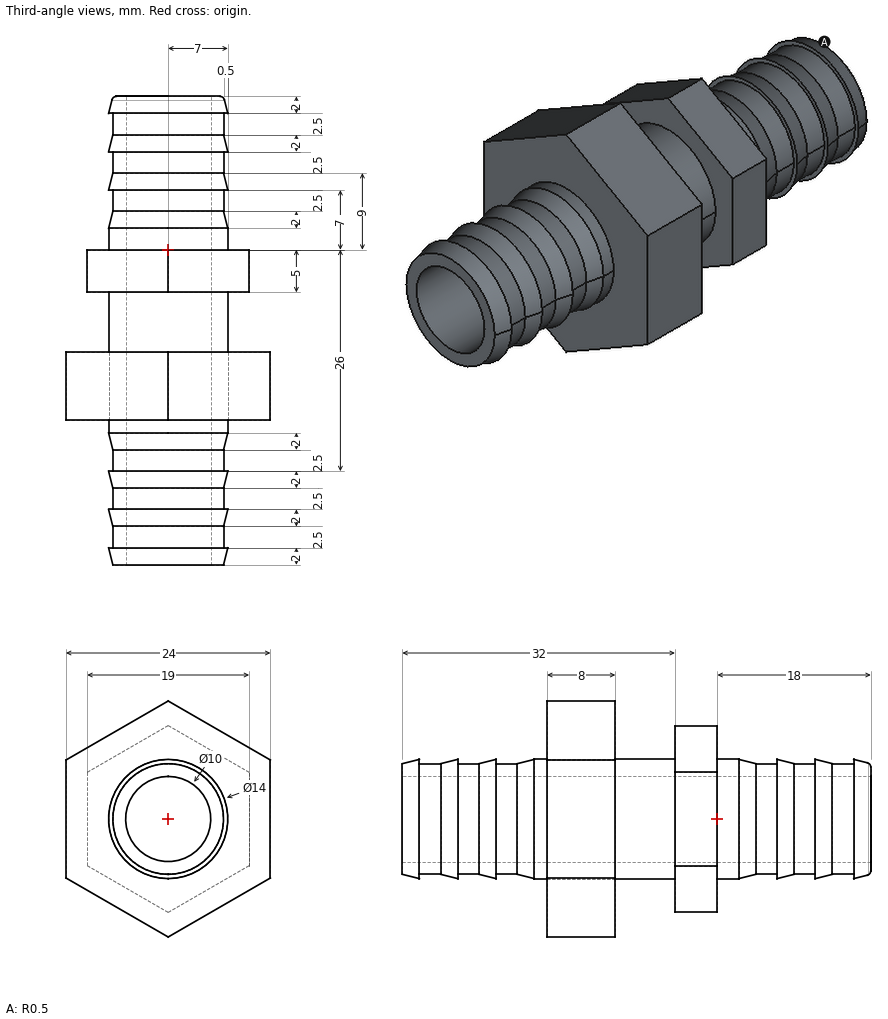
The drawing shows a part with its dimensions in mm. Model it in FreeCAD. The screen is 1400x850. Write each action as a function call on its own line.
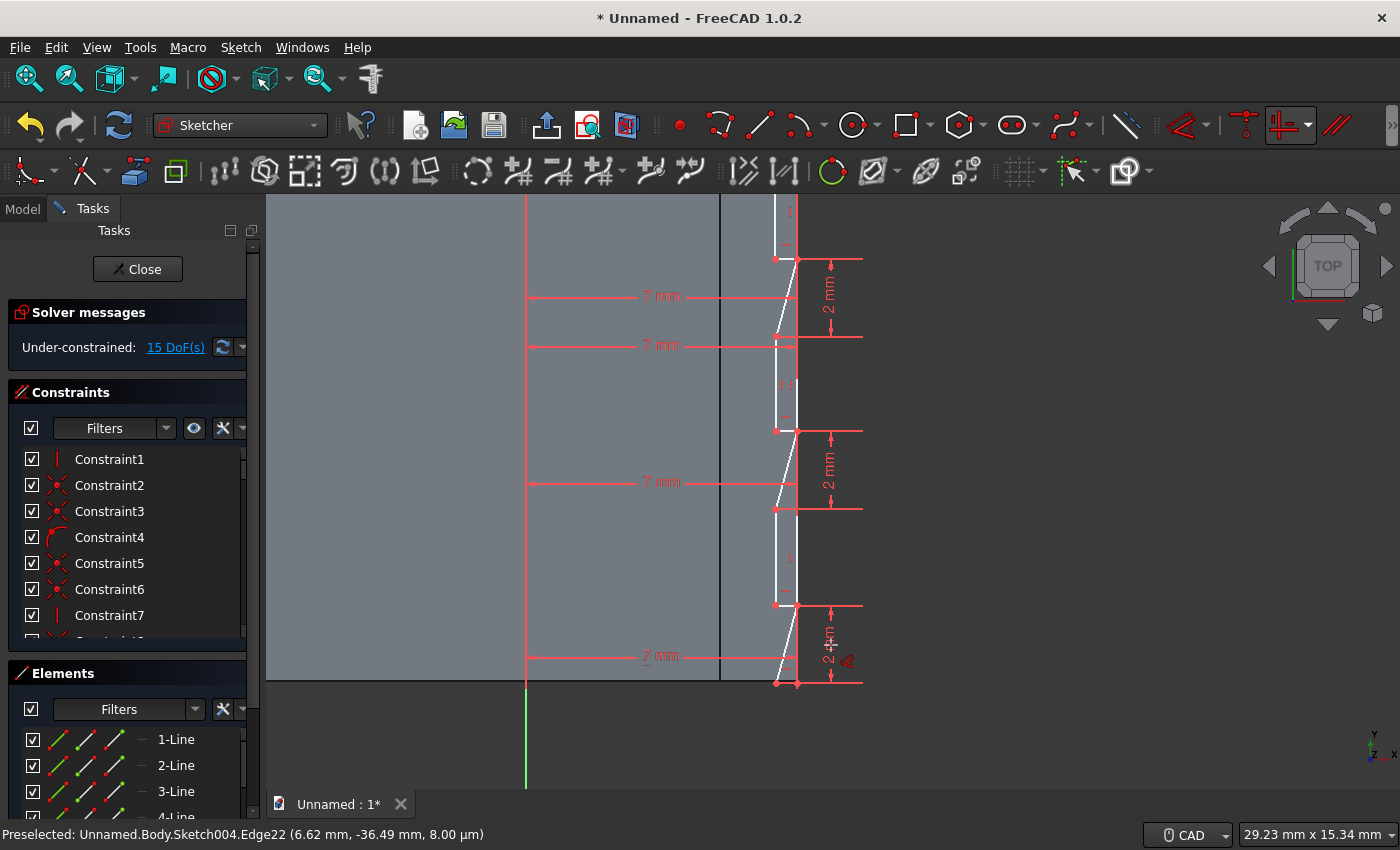
scroll(785, 665, down, 9)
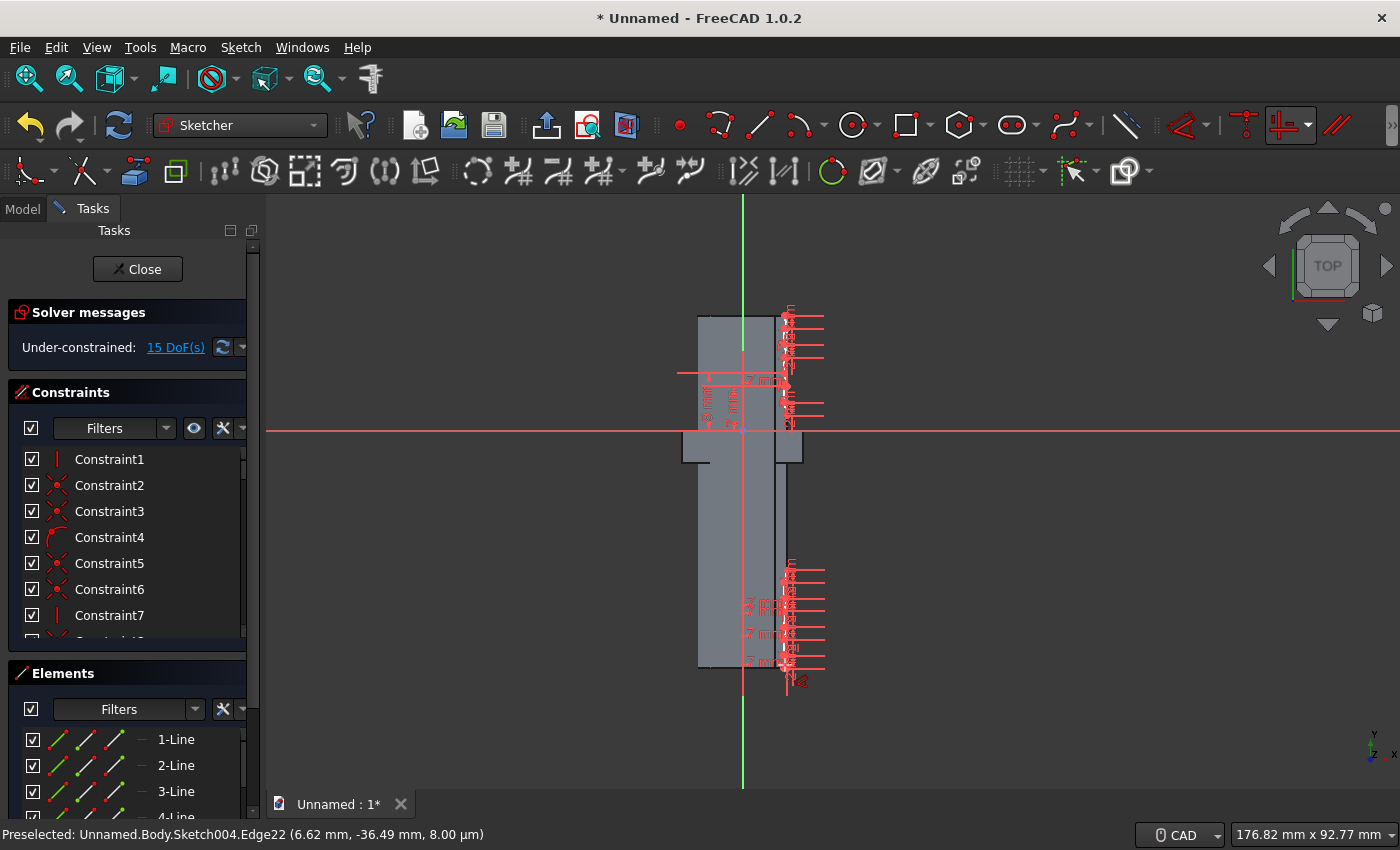
scroll(786, 316, up, 13)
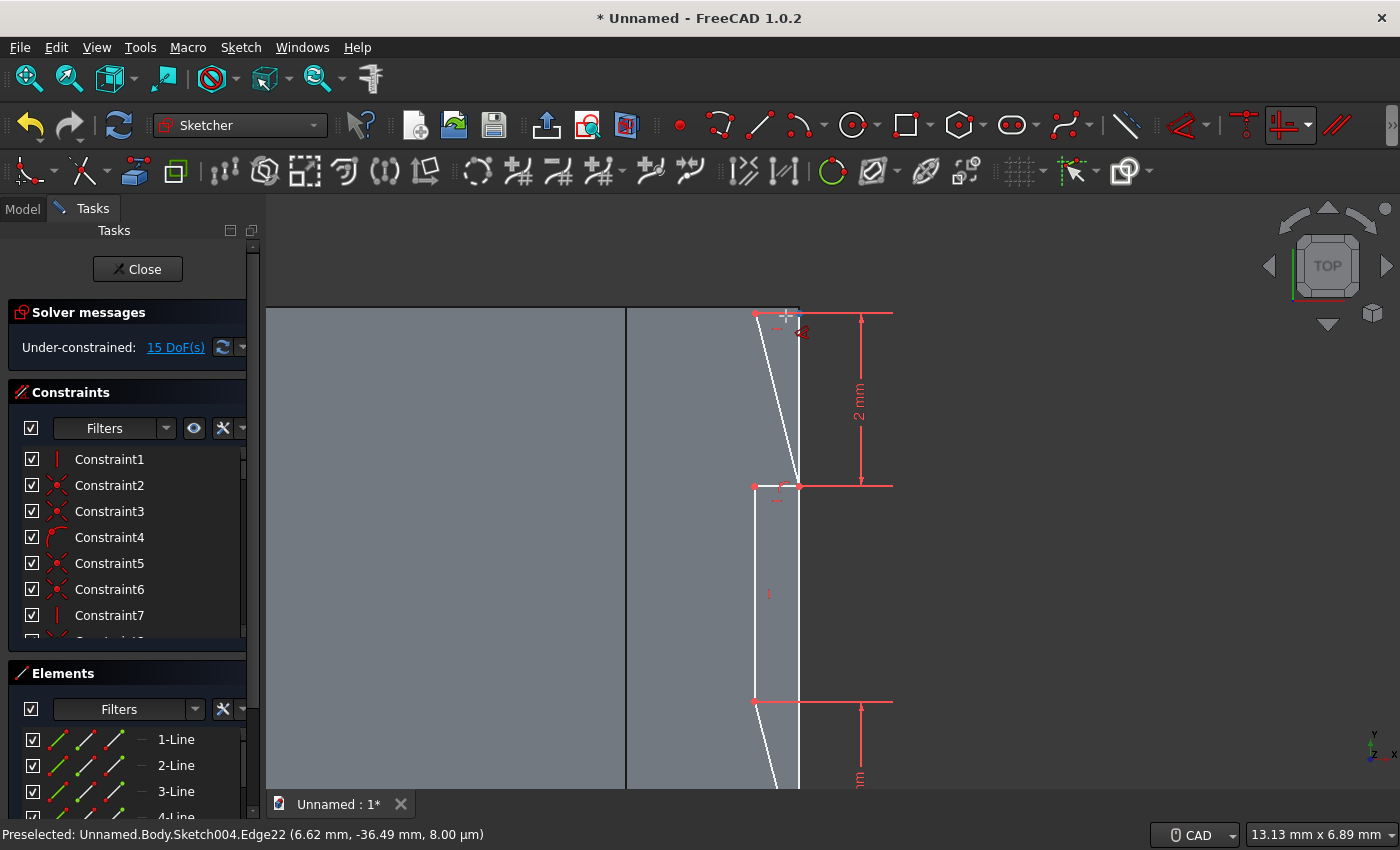
click(777, 313)
click(777, 279)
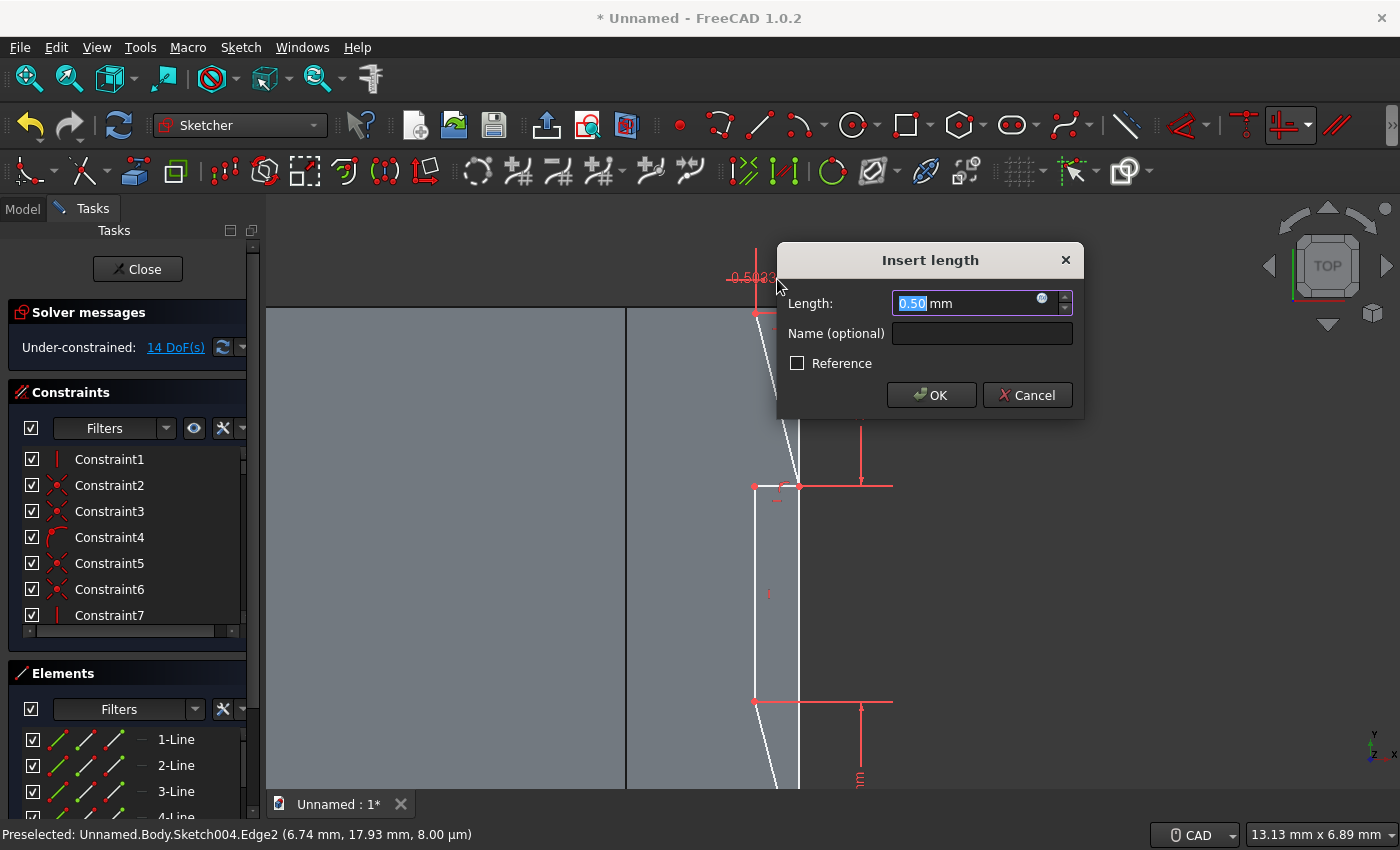
text(0.5)
key(Return)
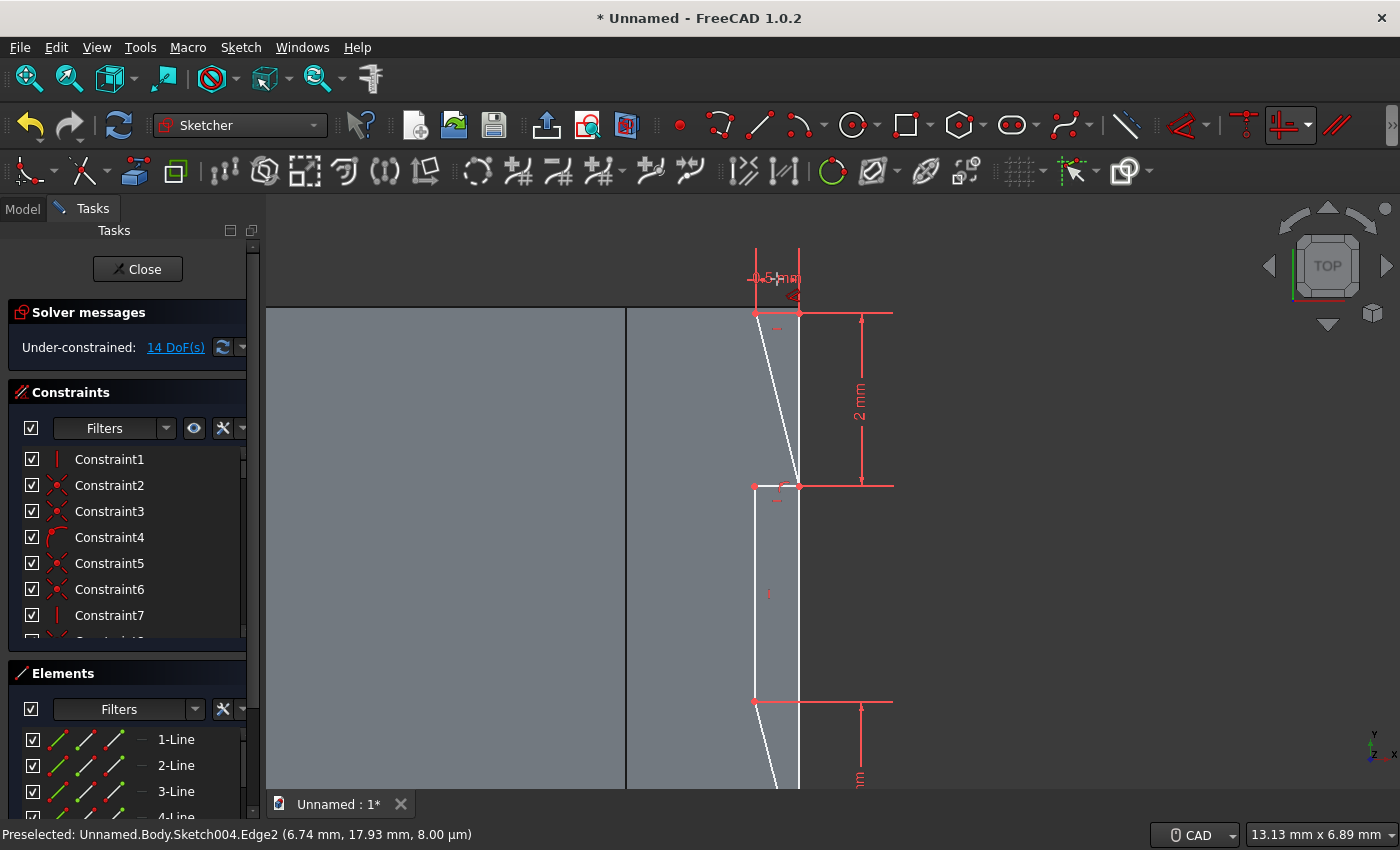
click(786, 486)
click(777, 452)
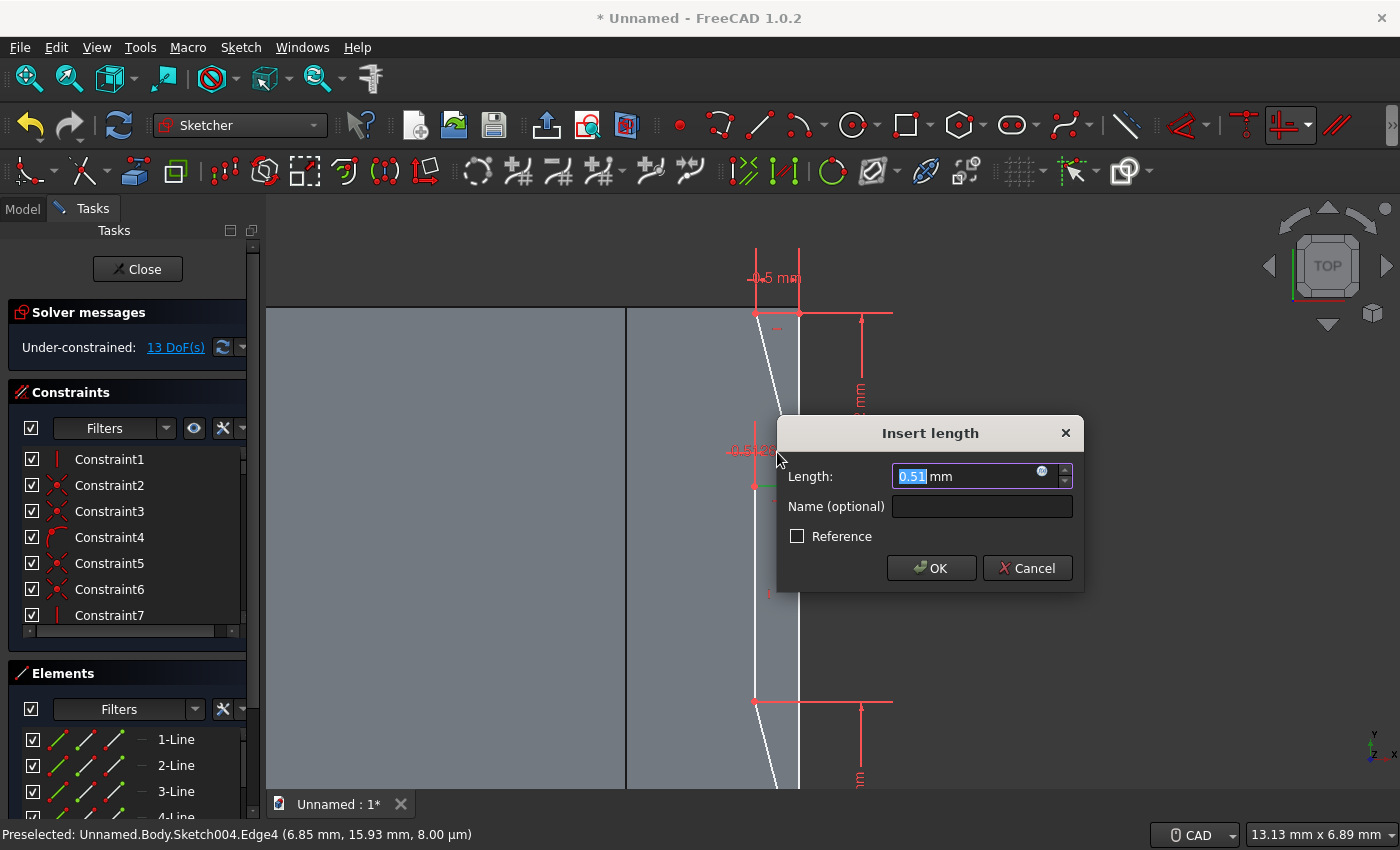
text(0.5)
key(Return)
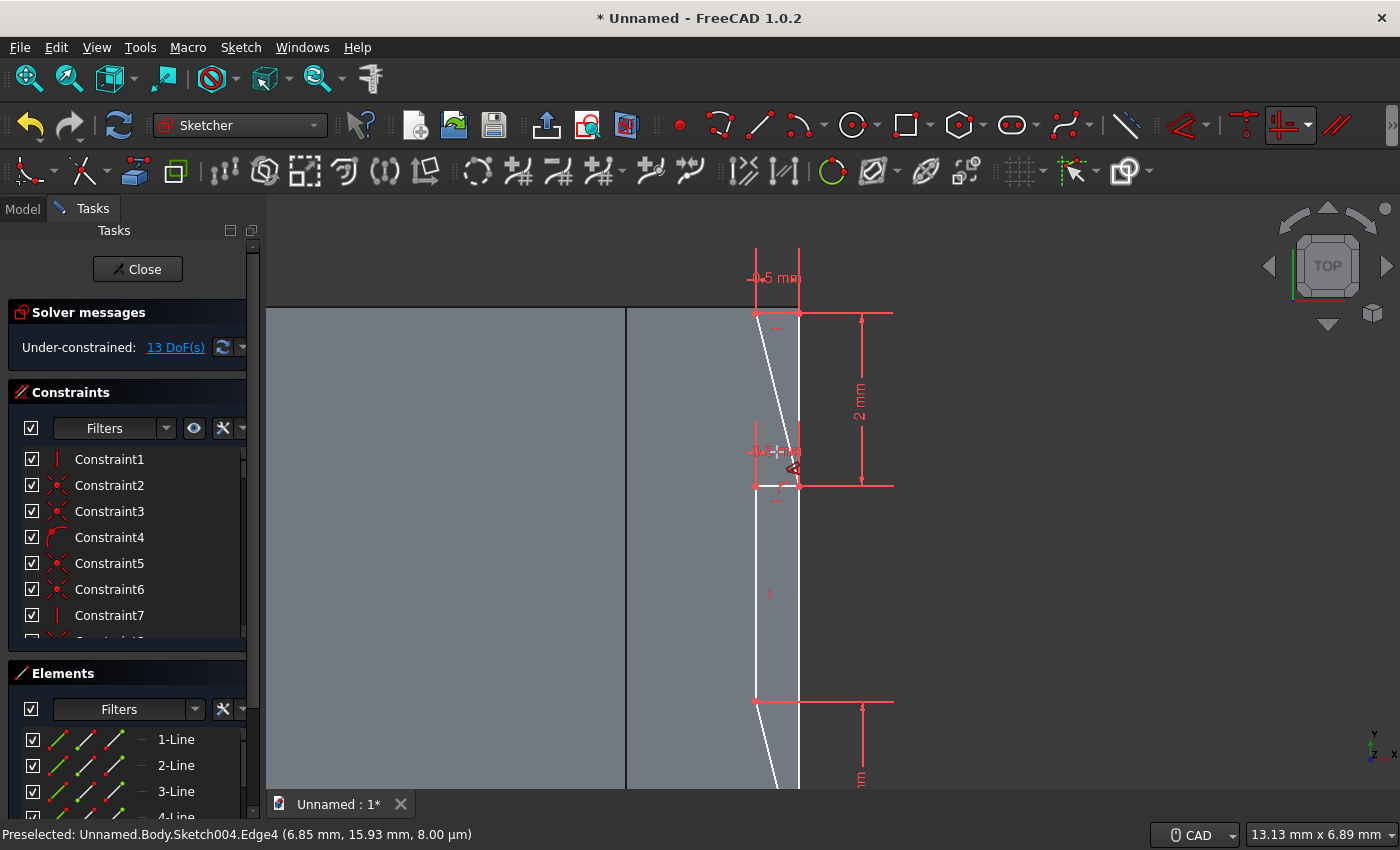
scroll(786, 316, down, 13)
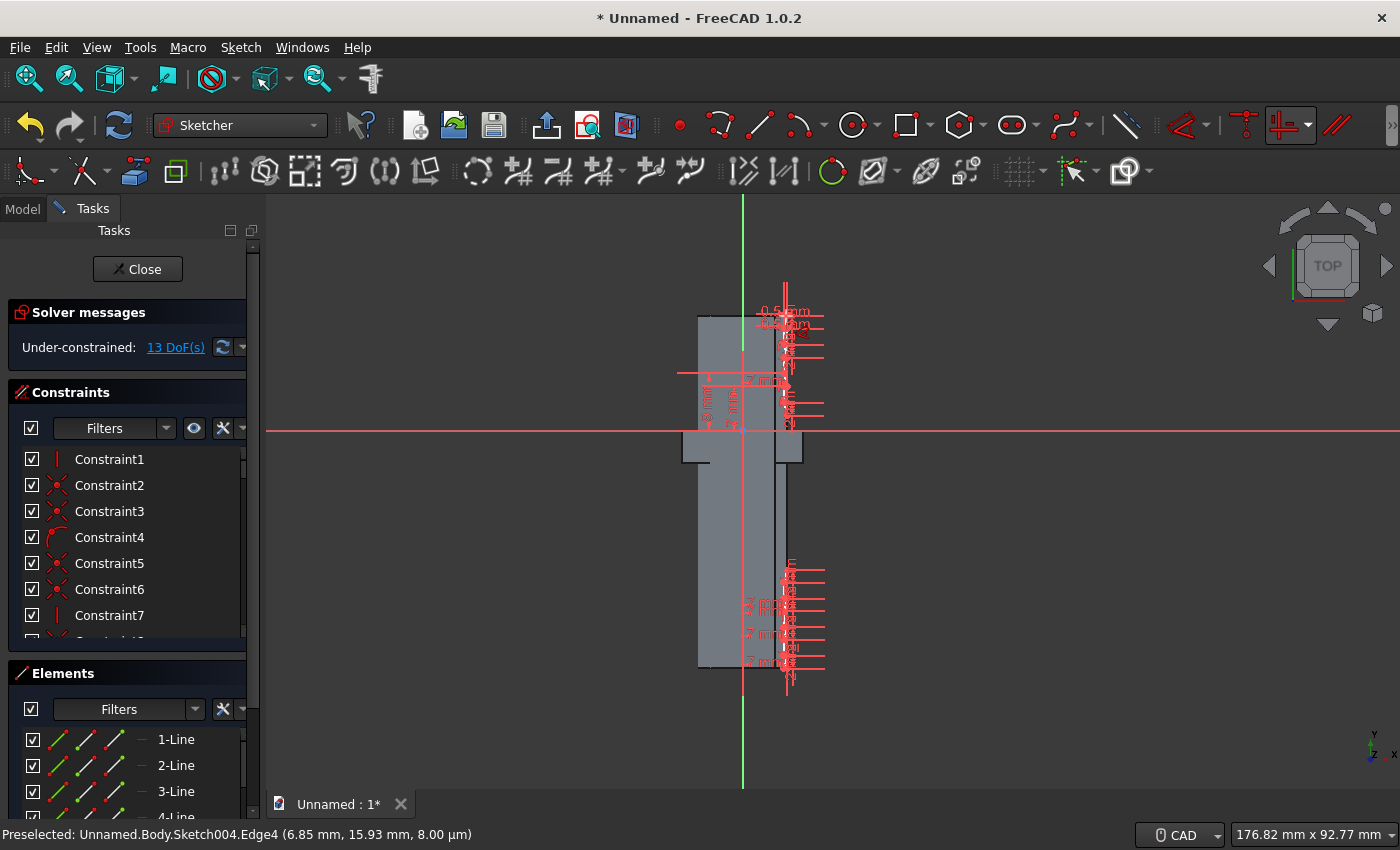
scroll(784, 334, up, 8)